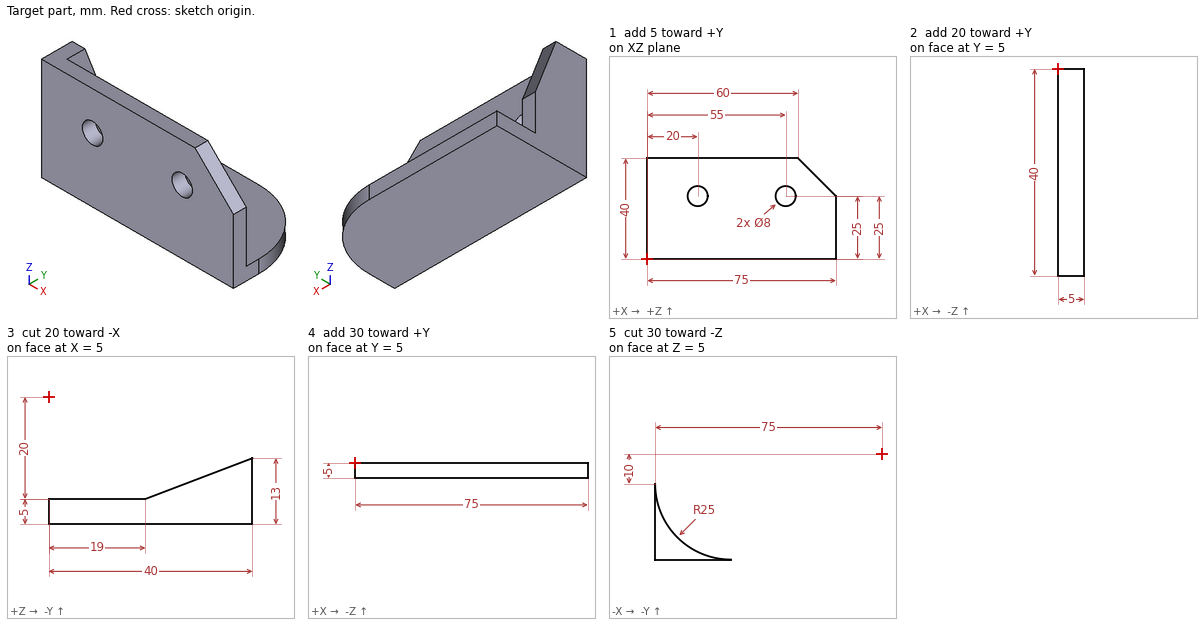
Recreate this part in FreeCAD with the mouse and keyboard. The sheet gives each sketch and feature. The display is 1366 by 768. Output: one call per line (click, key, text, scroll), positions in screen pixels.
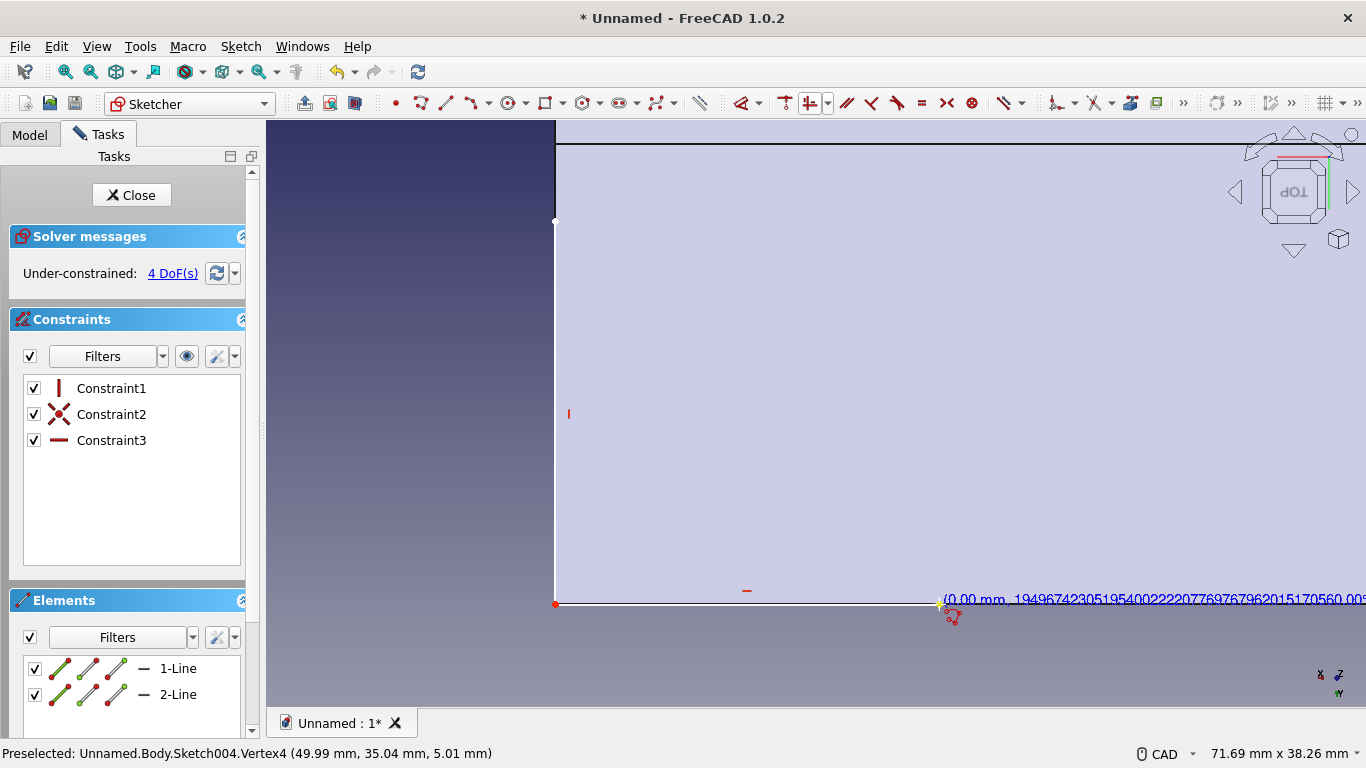
click(470, 104)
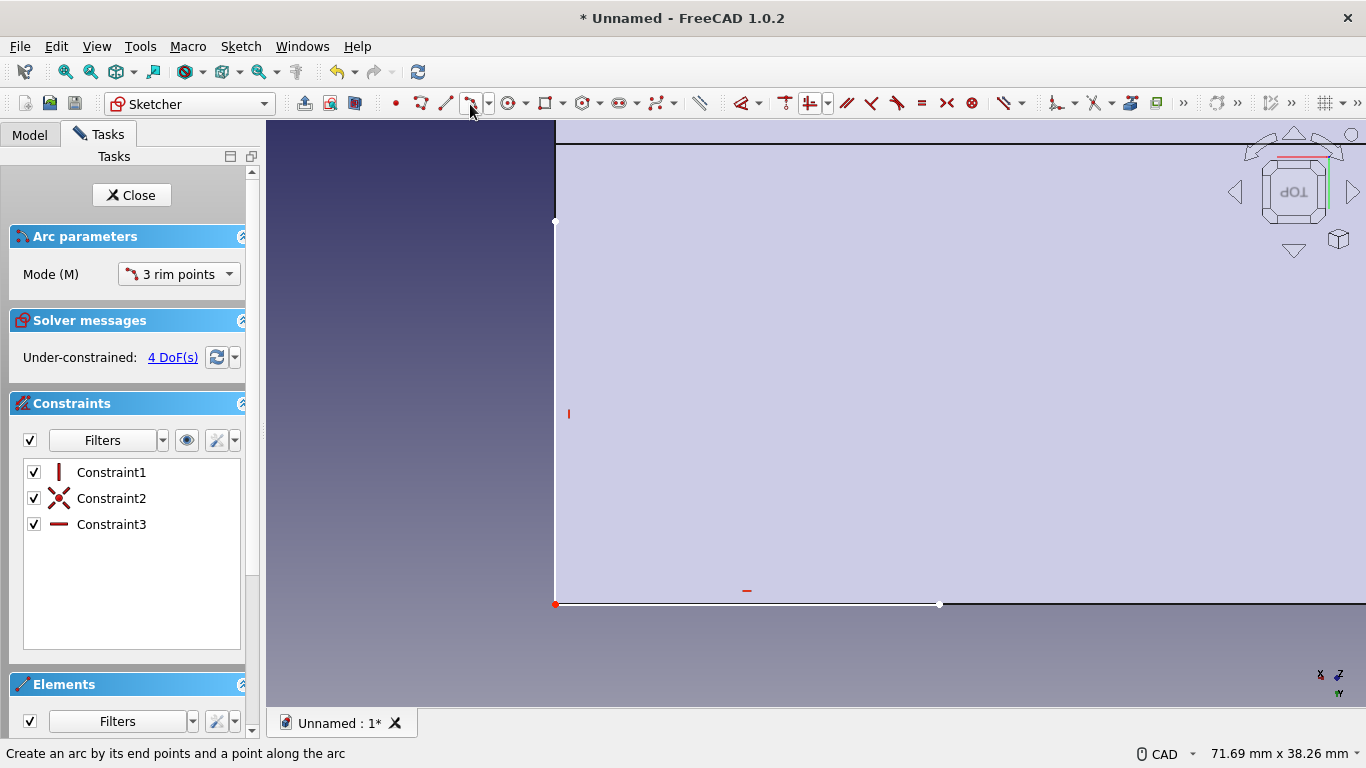
click(939, 605)
click(555, 222)
click(668, 492)
key(Escape)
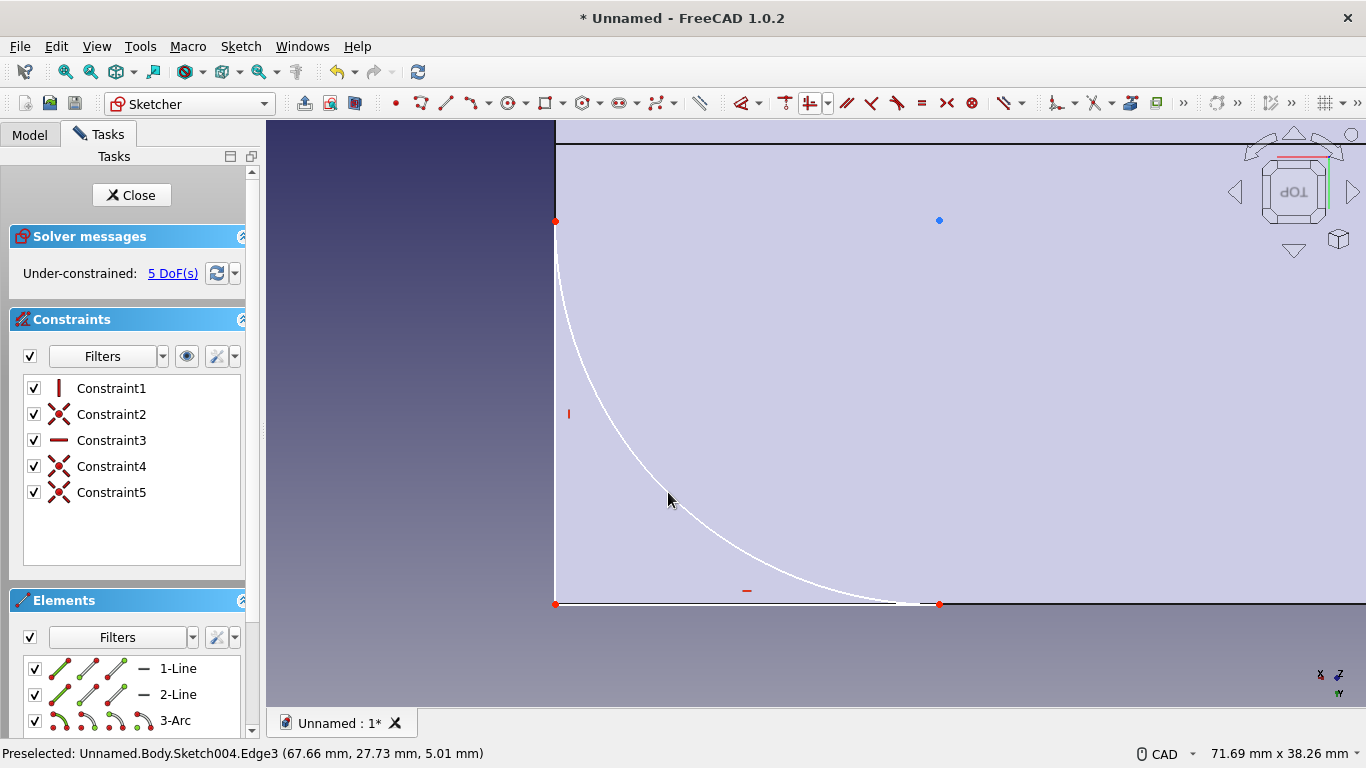
click(555, 337)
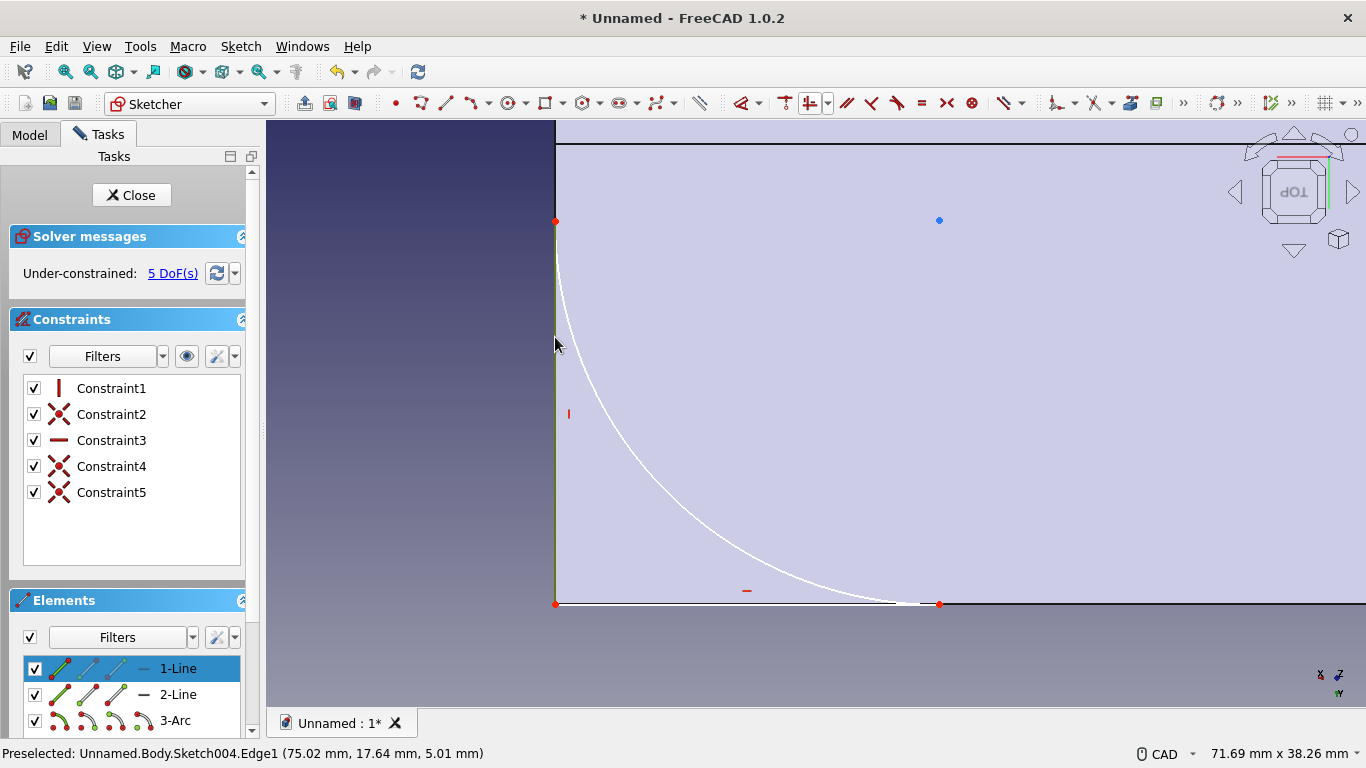
click(597, 396)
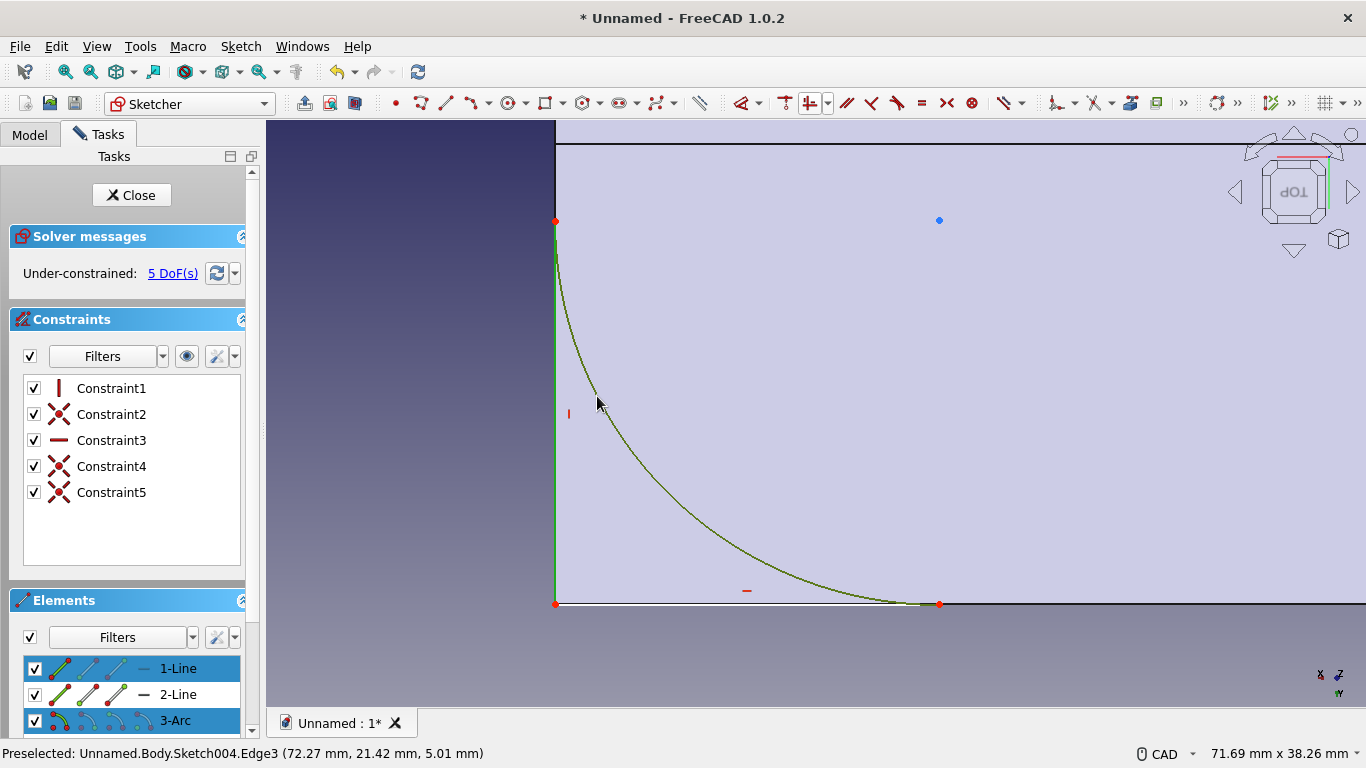
click(897, 104)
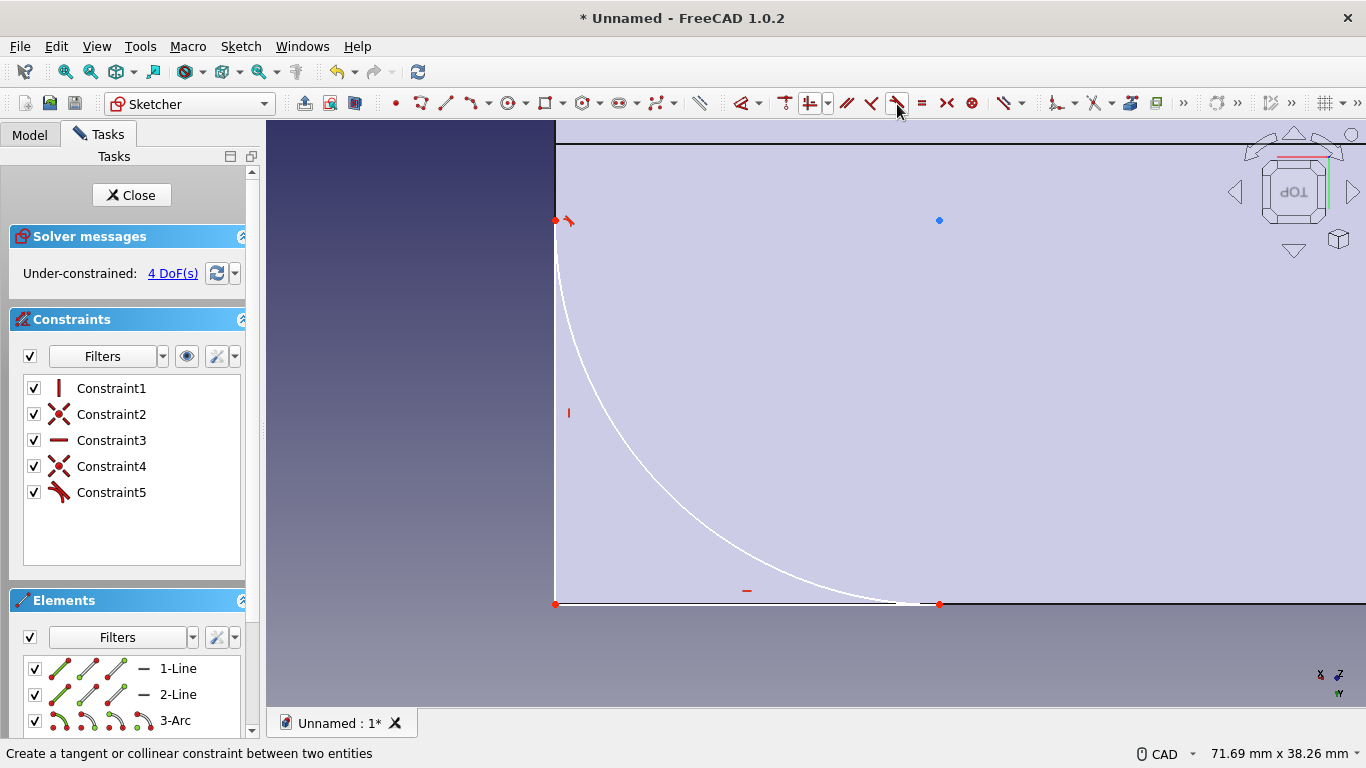
click(670, 605)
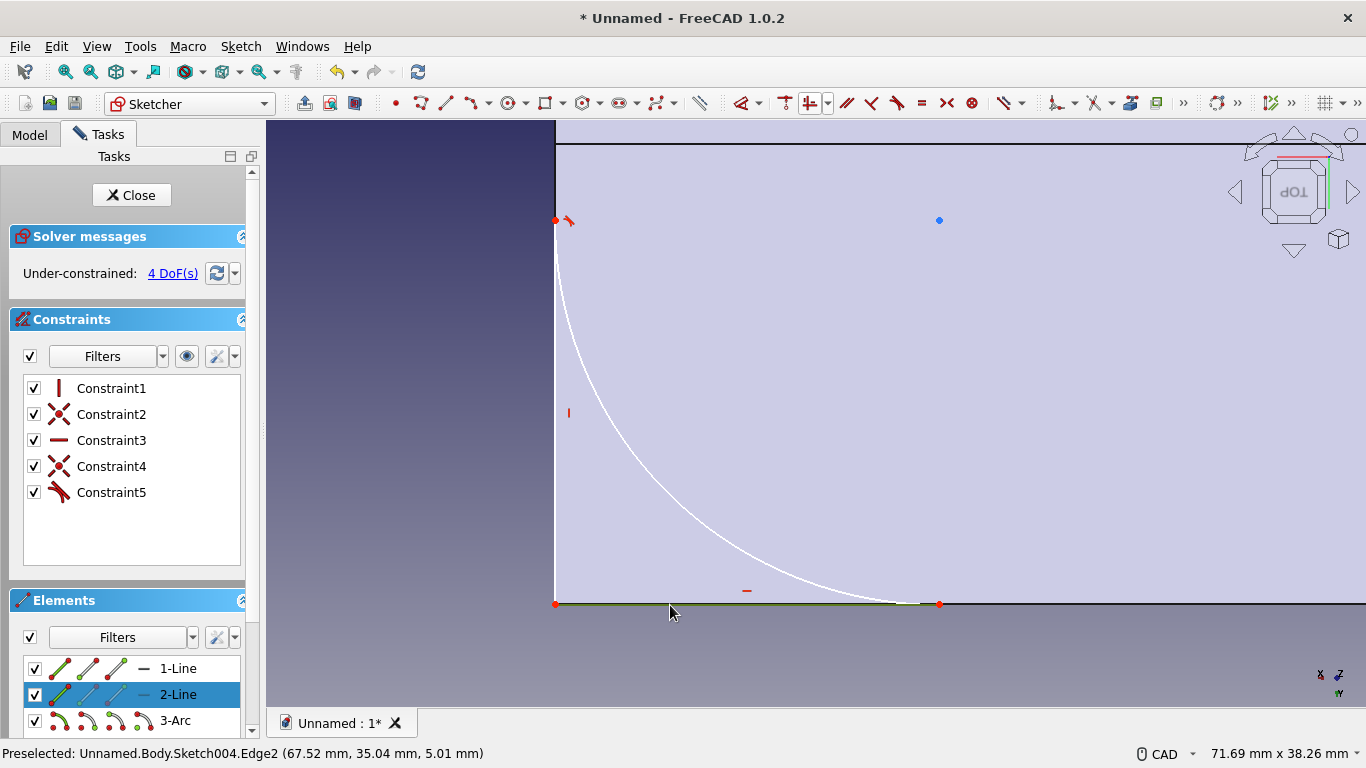
click(597, 395)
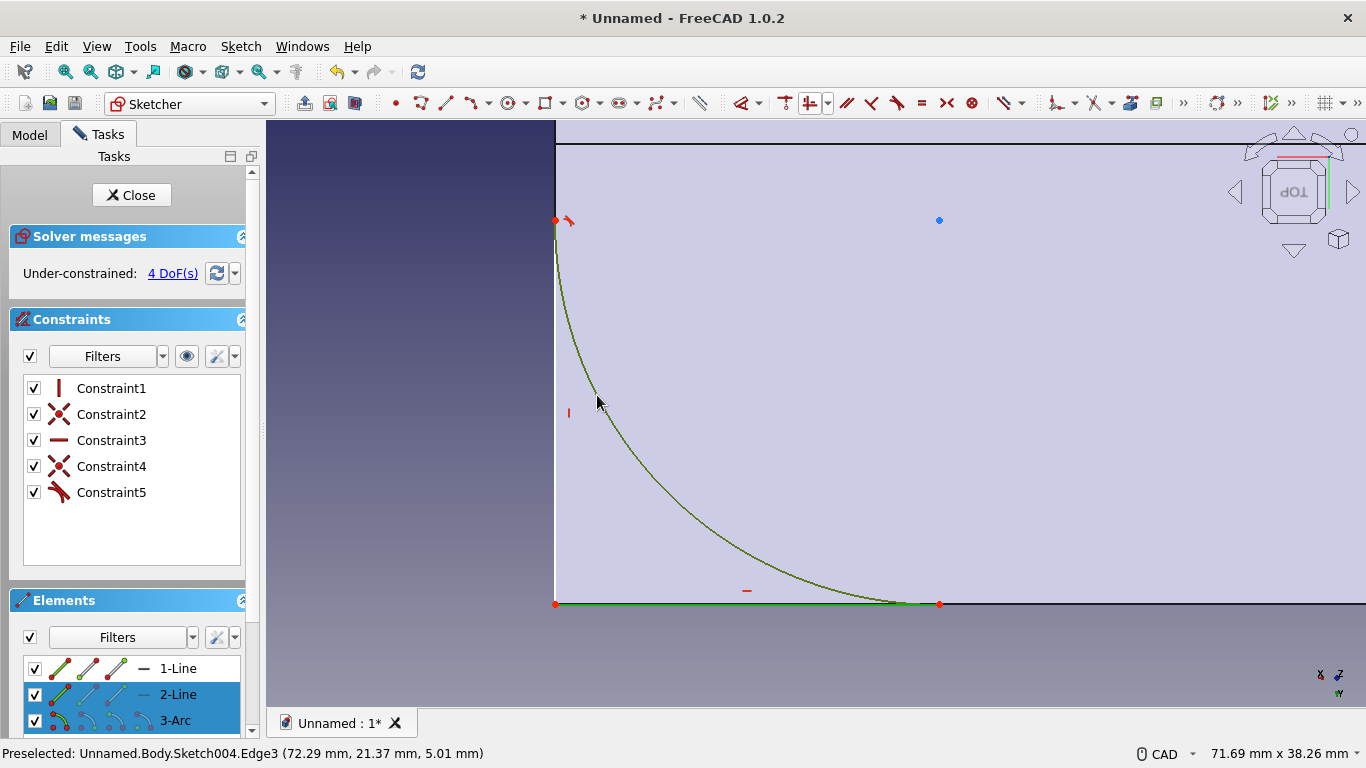
click(897, 104)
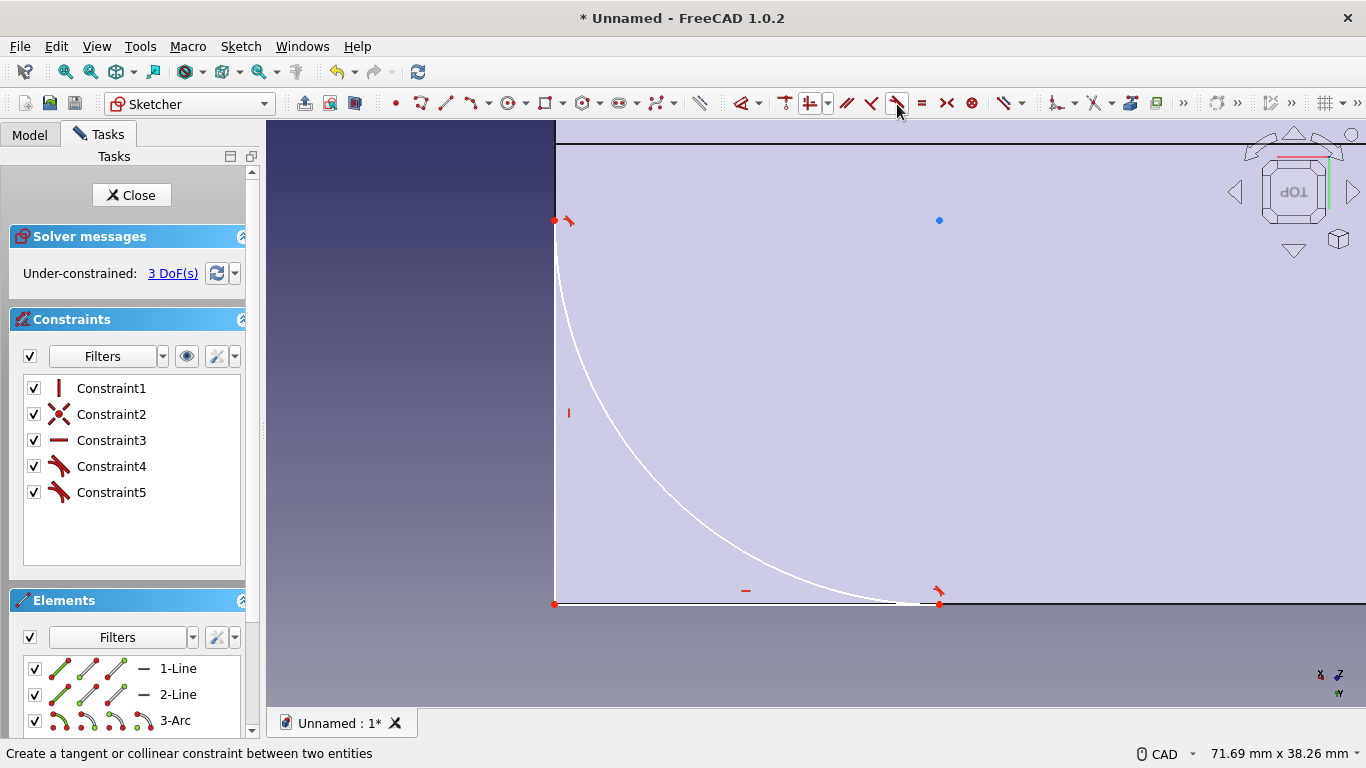
click(740, 104)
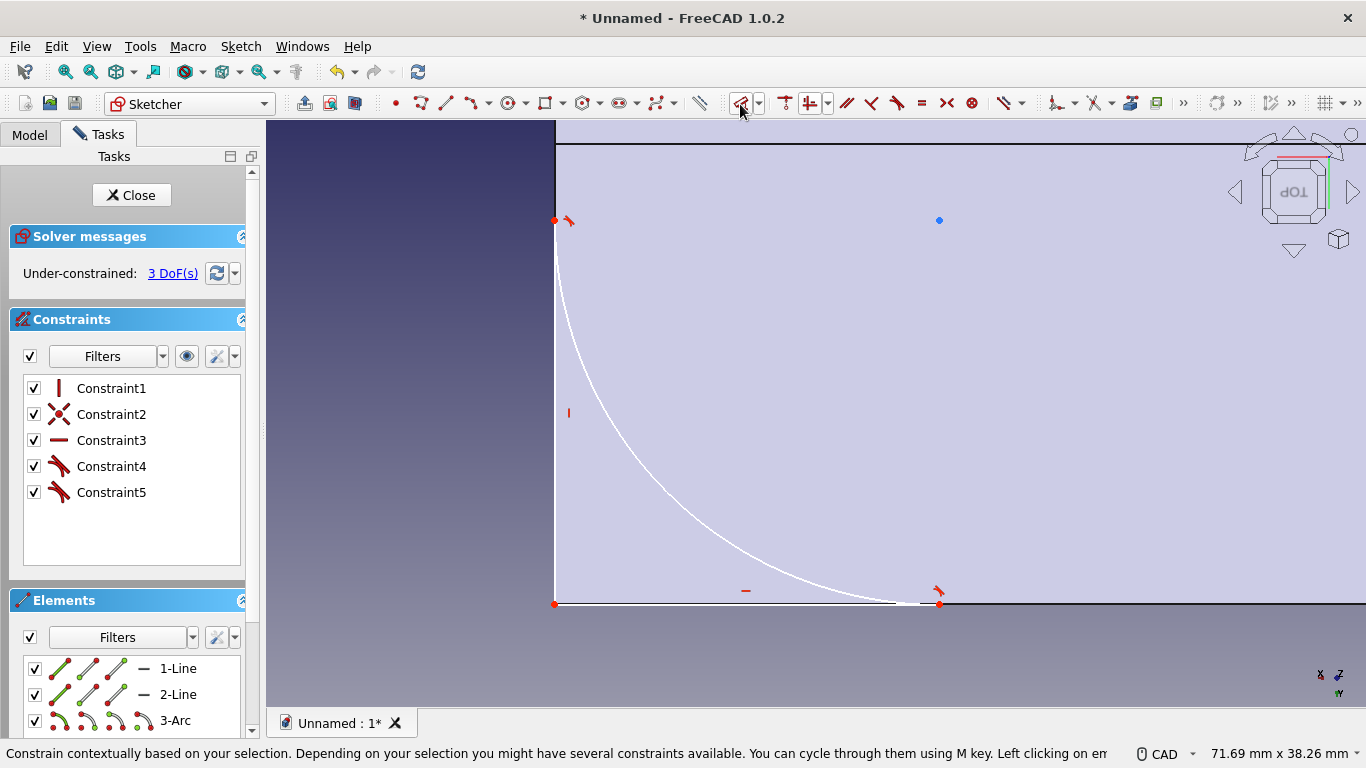
click(597, 395)
click(568, 410)